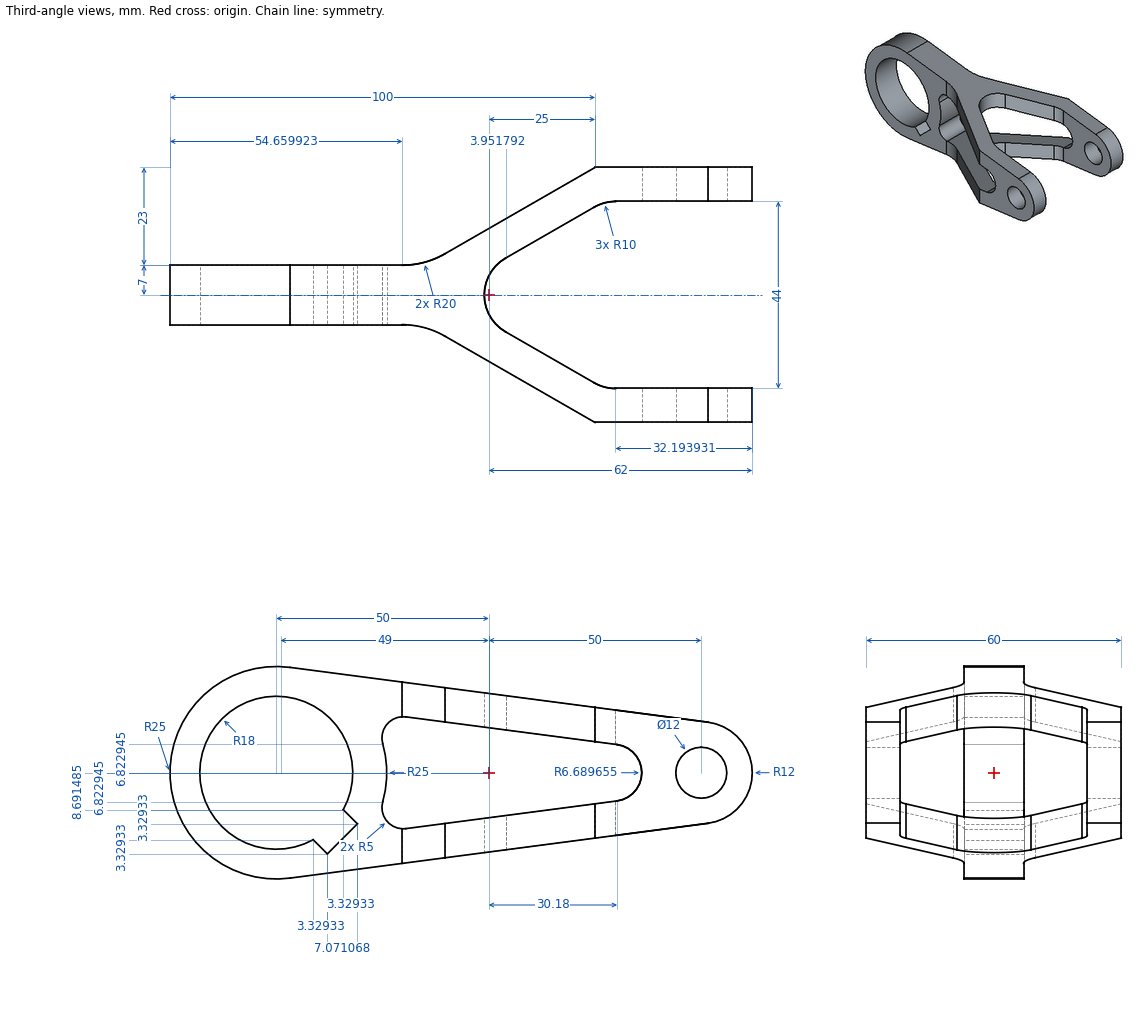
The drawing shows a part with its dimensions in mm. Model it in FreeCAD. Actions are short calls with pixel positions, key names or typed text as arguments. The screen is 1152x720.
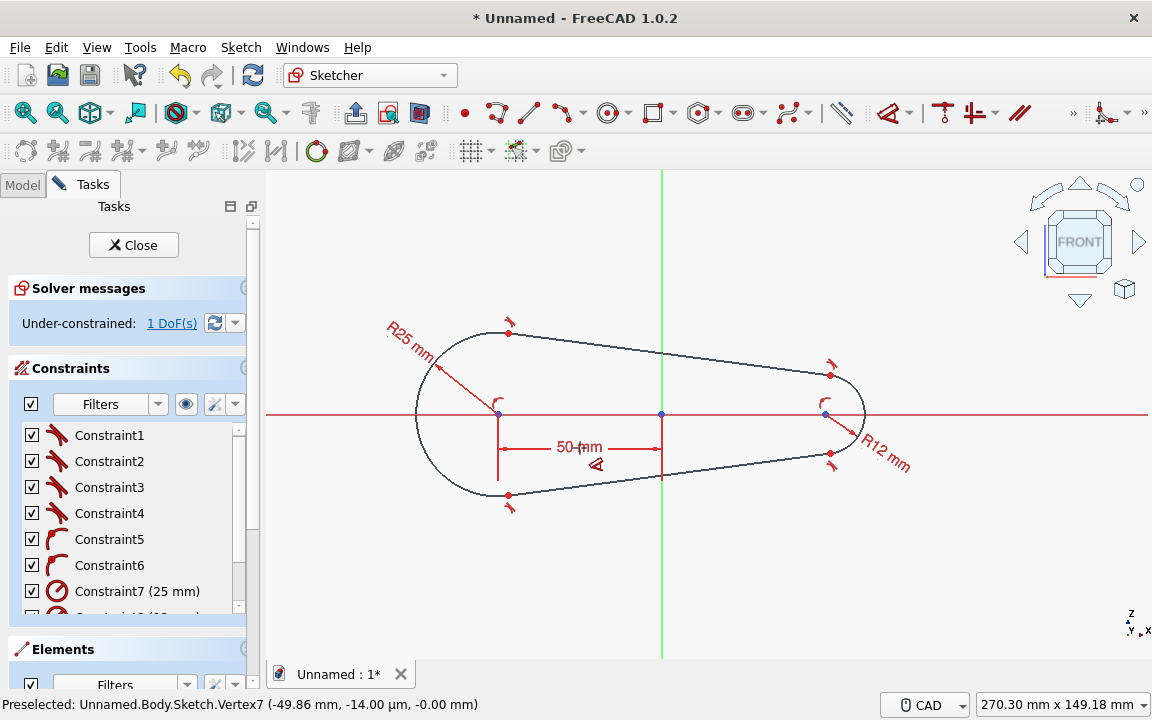
click(825, 414)
click(744, 448)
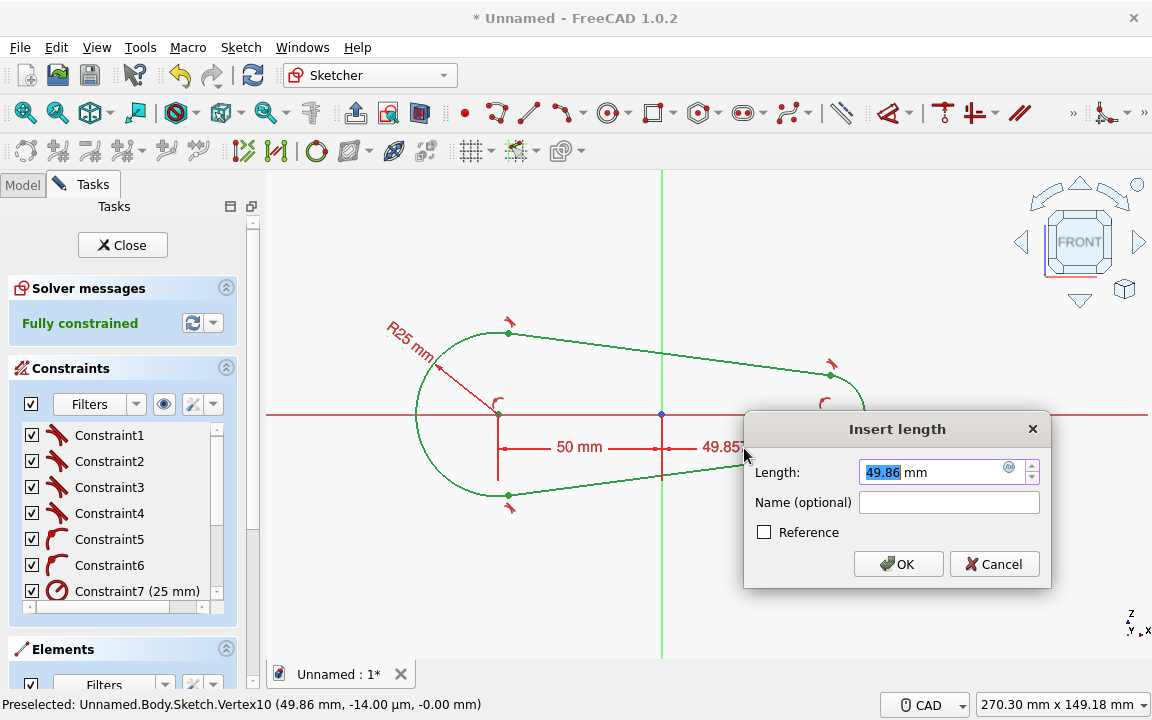
text(50)
key(Return)
key(Escape)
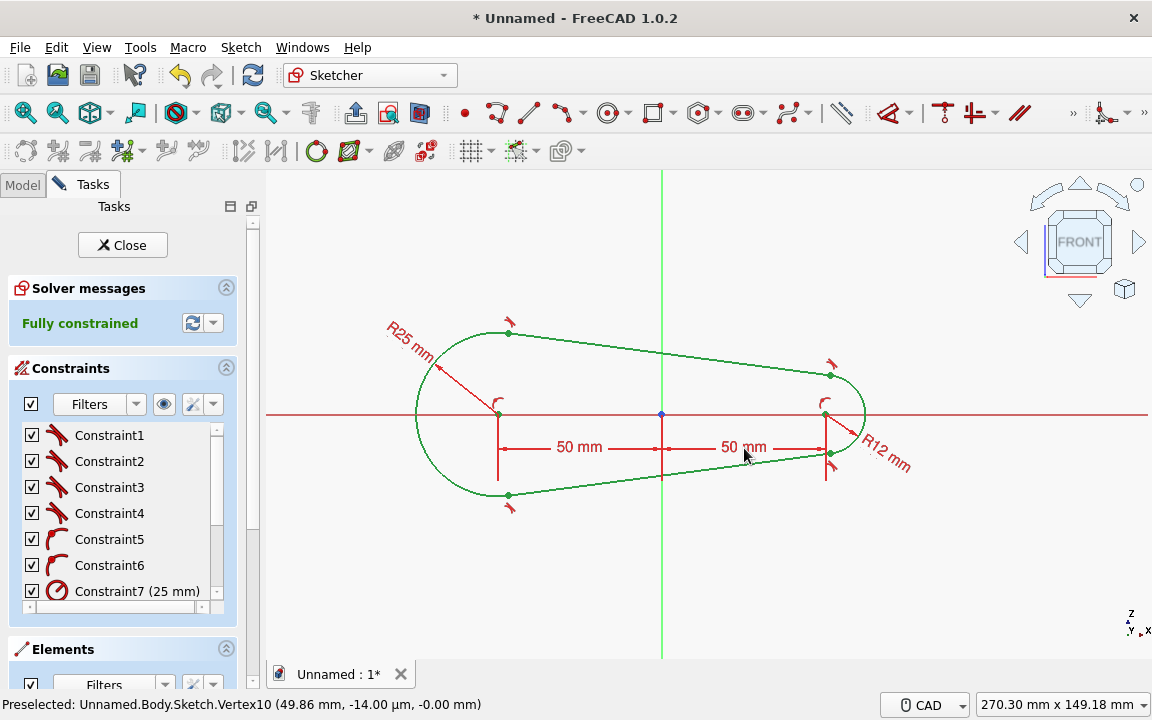
click(123, 245)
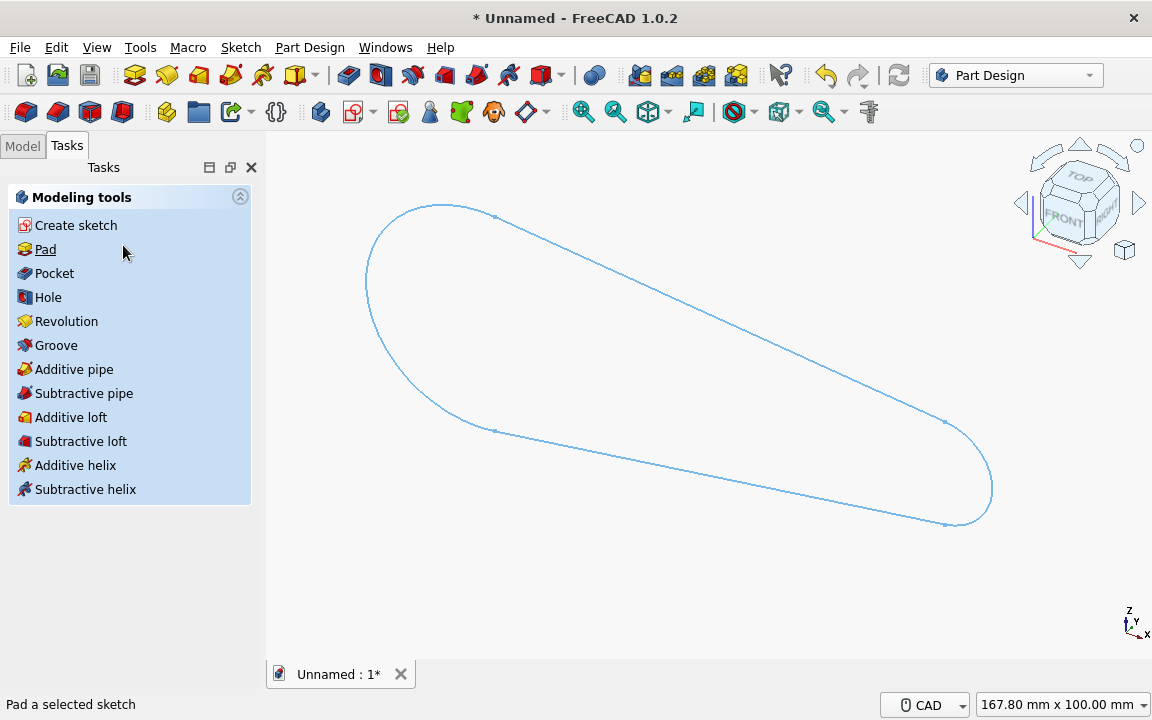
click(136, 76)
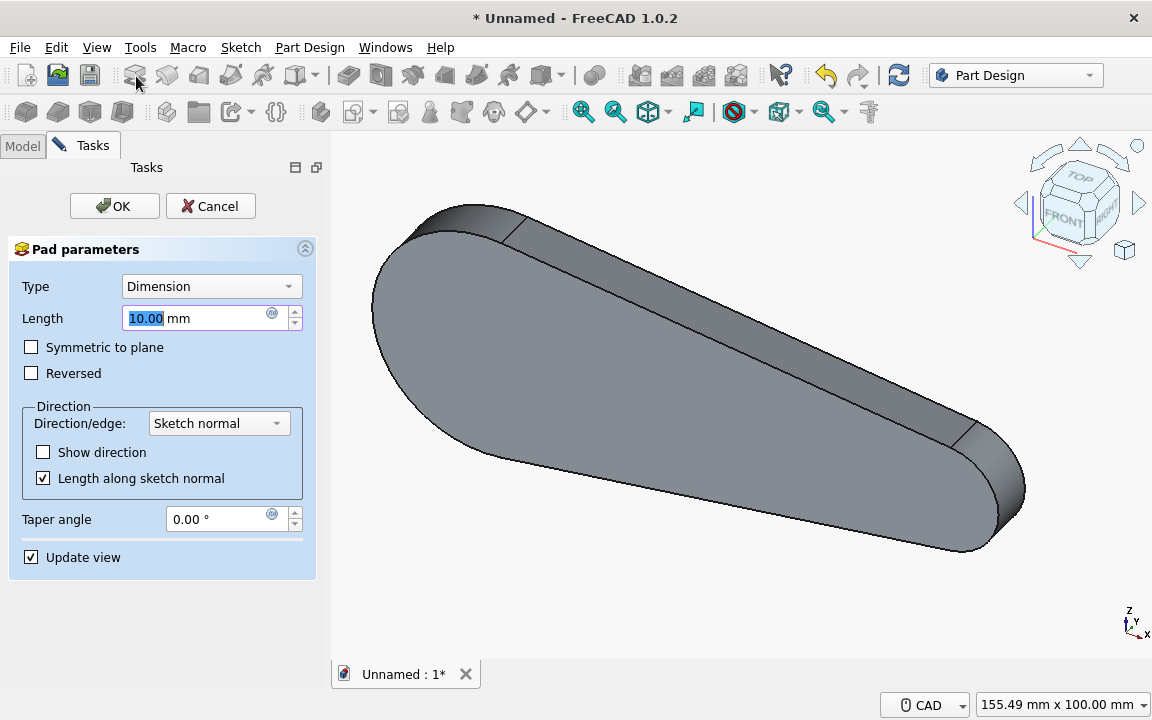
text(60)
key(Tab)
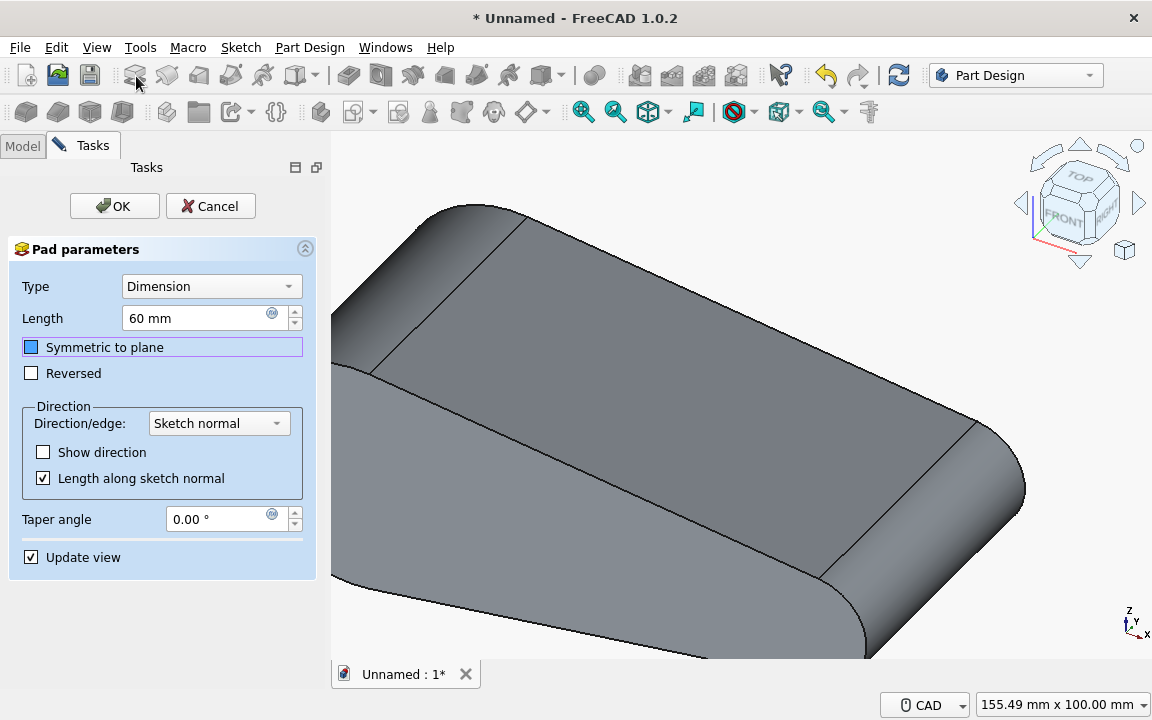
click(30, 347)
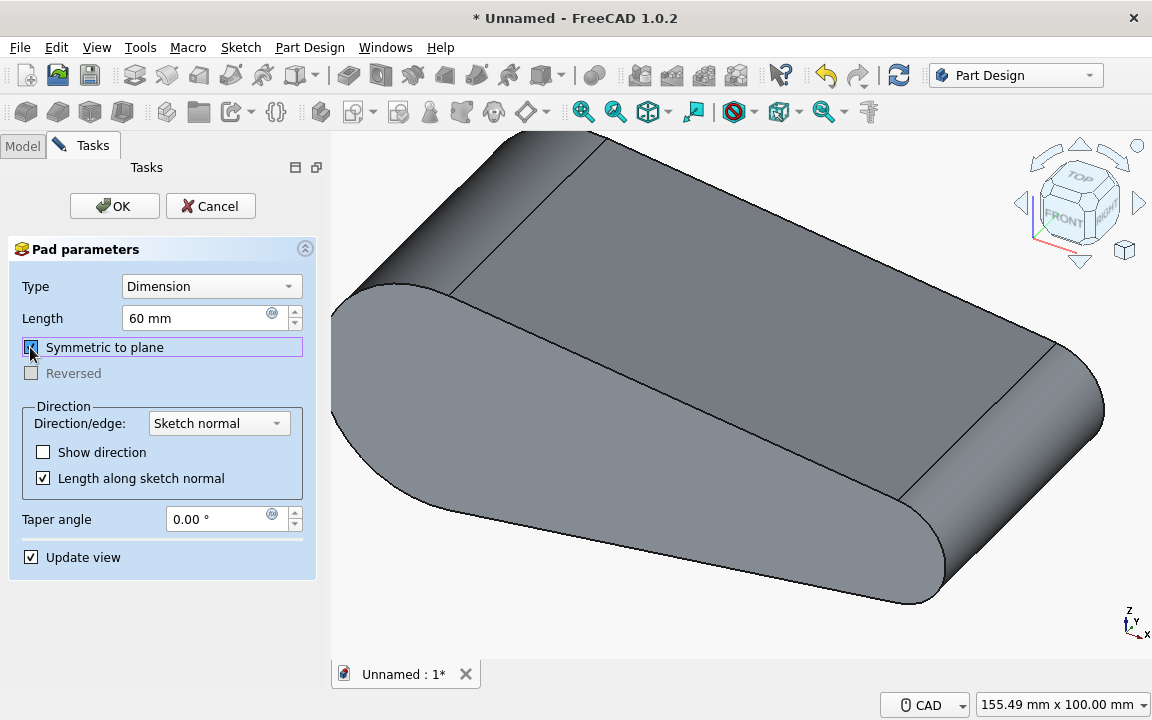
click(115, 206)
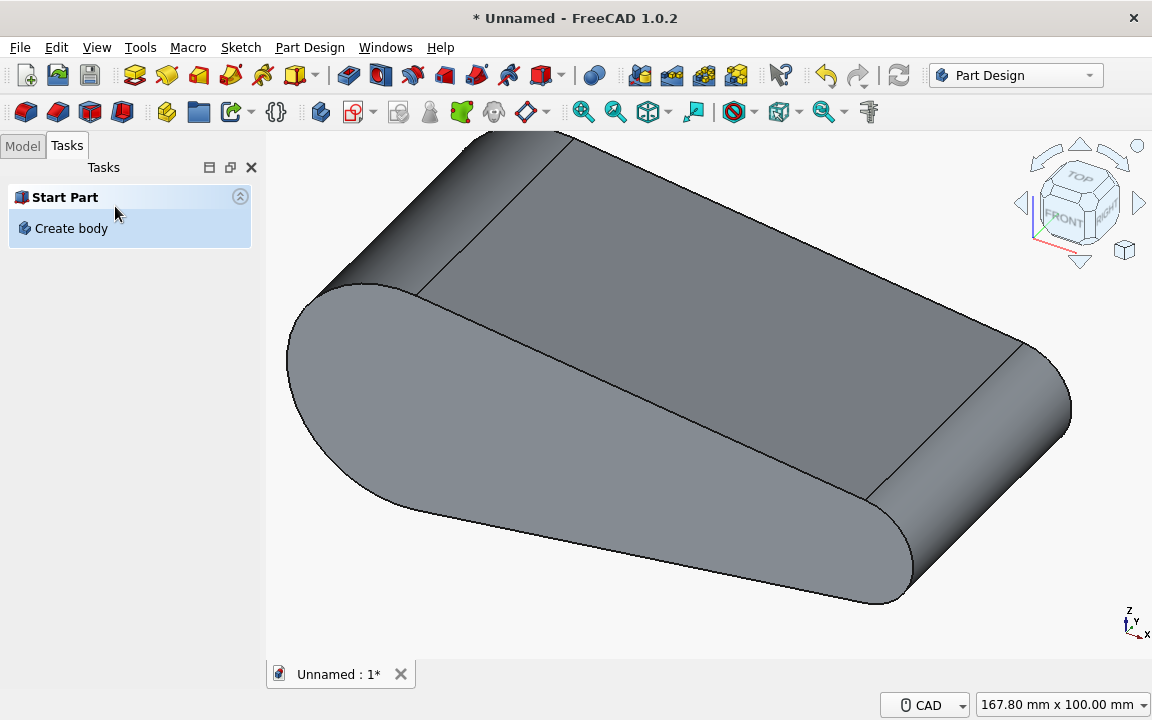
click(584, 112)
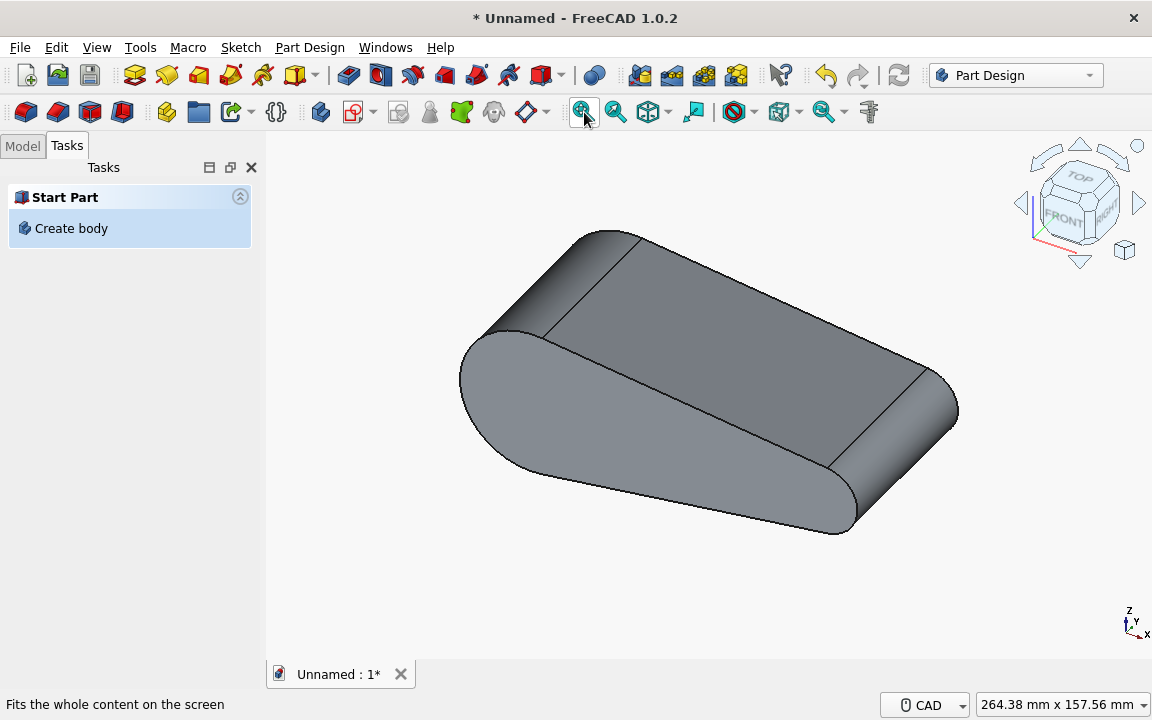
key(4)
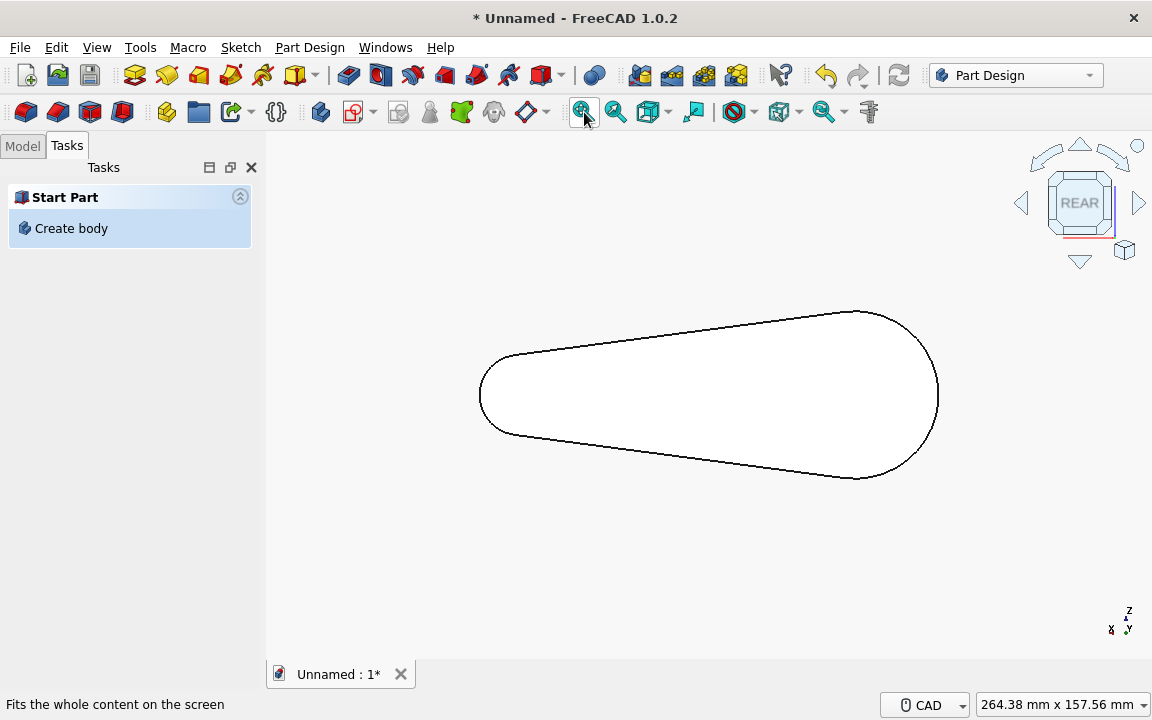
click(840, 394)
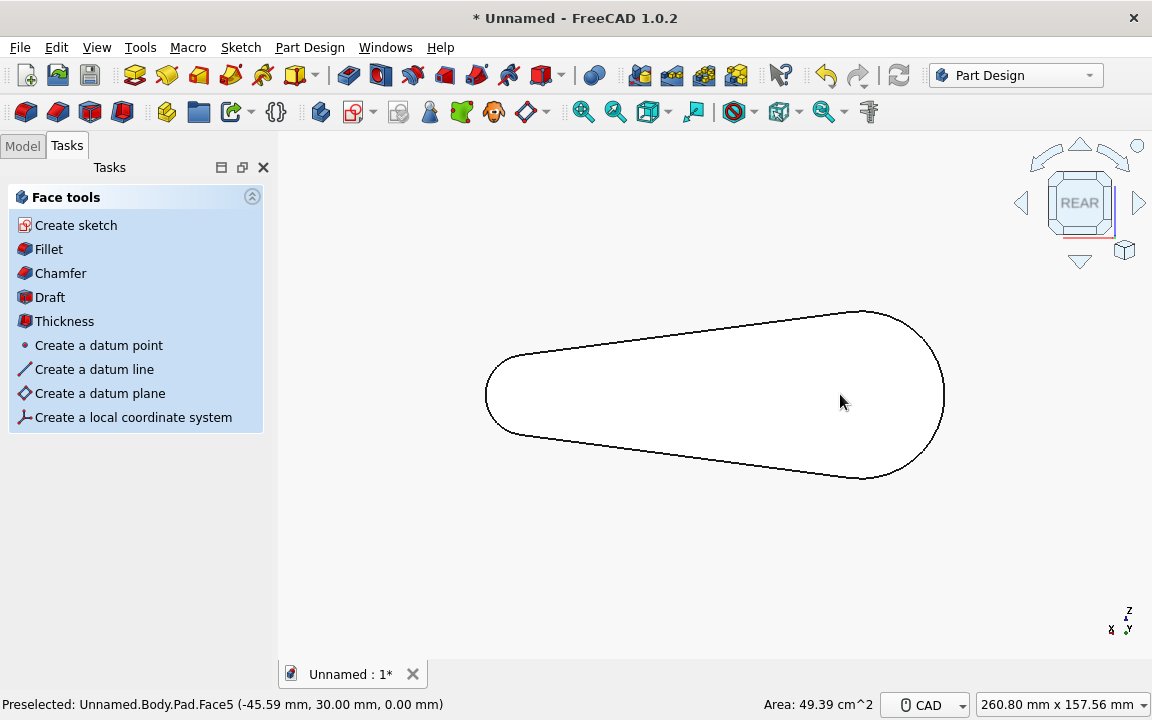
click(354, 112)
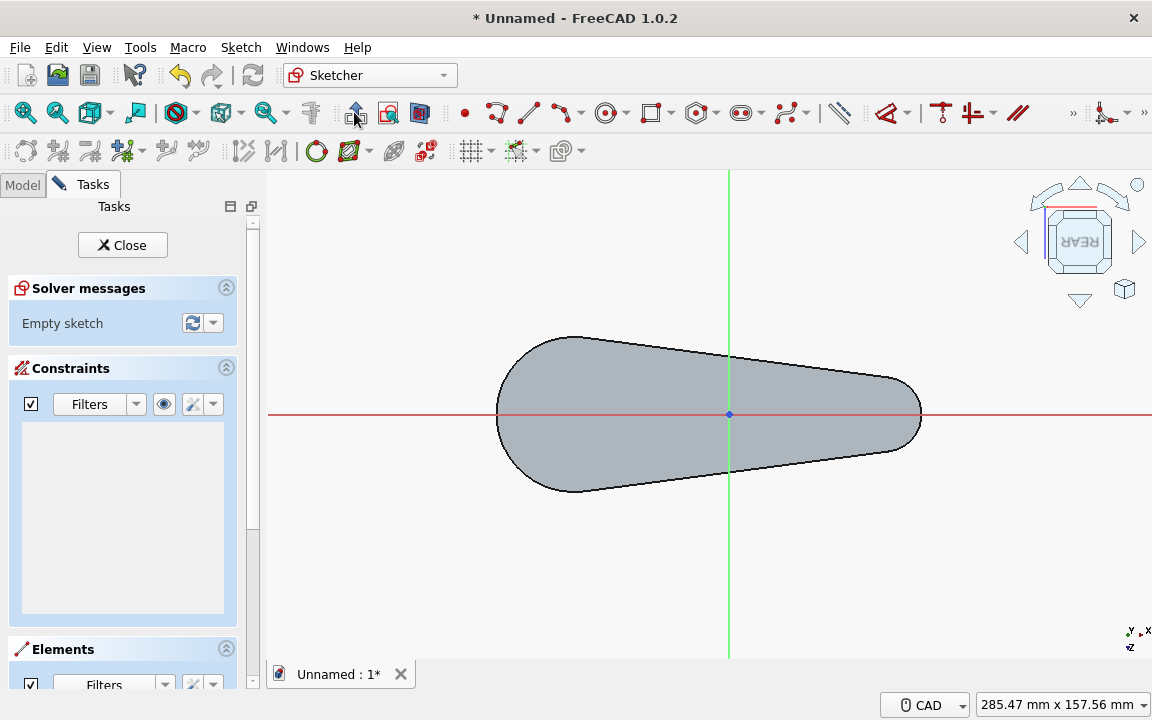
scroll(627, 399, up, 5)